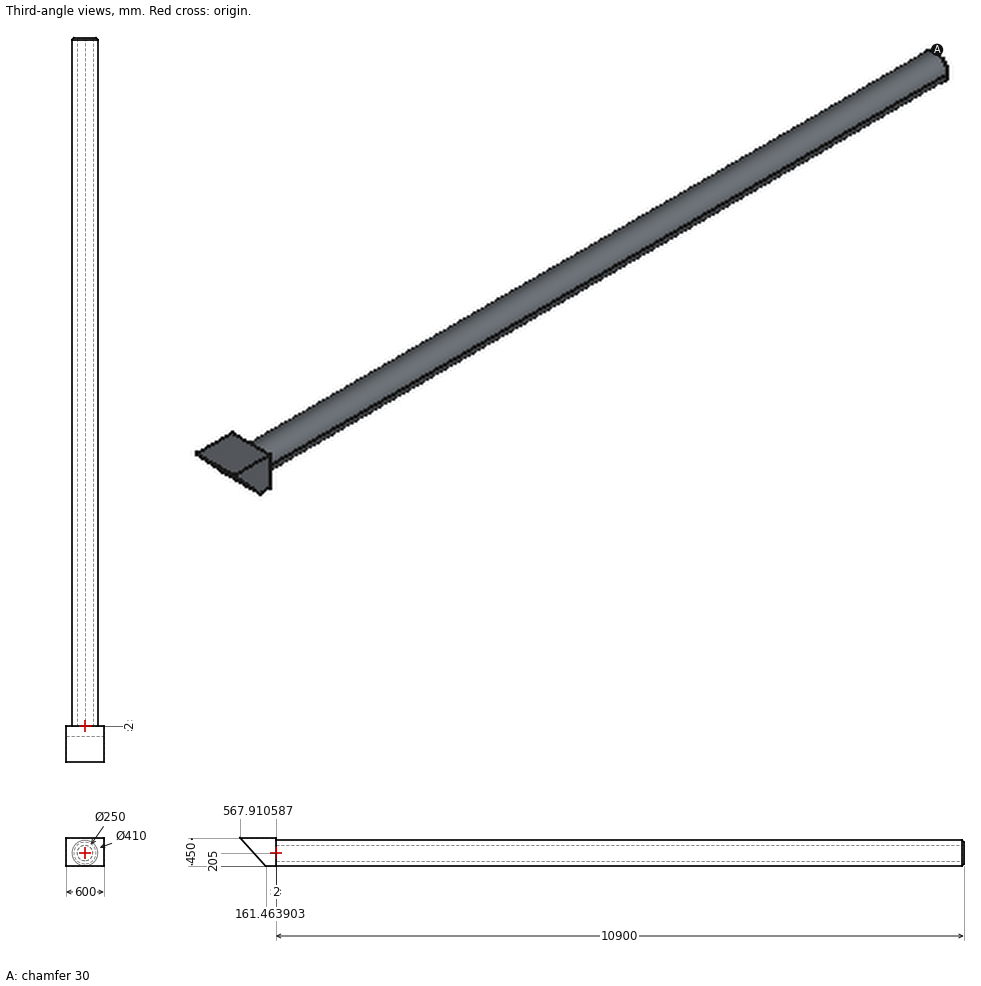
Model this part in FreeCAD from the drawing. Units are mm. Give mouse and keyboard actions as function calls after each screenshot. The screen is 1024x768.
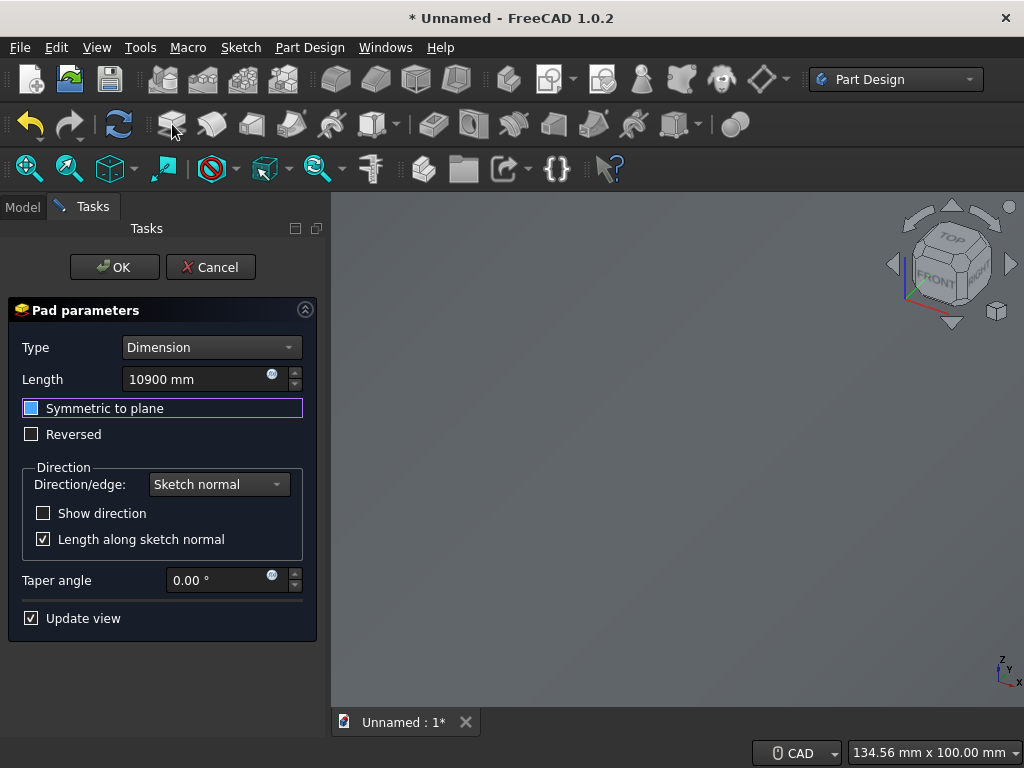
click(30, 434)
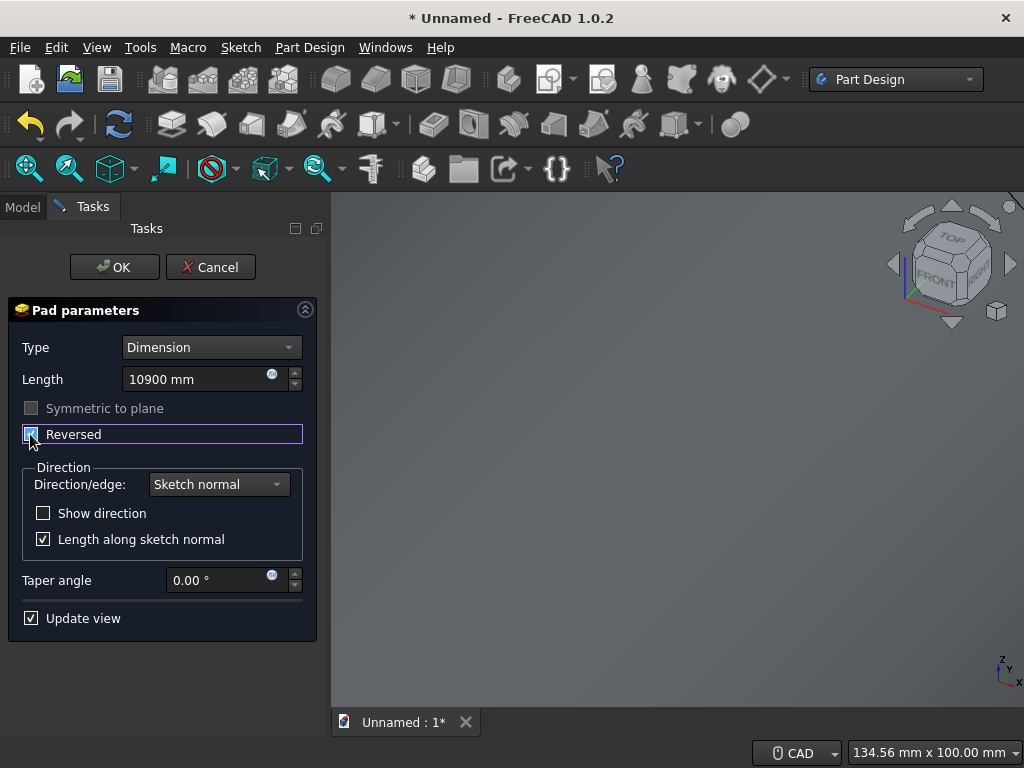
click(115, 267)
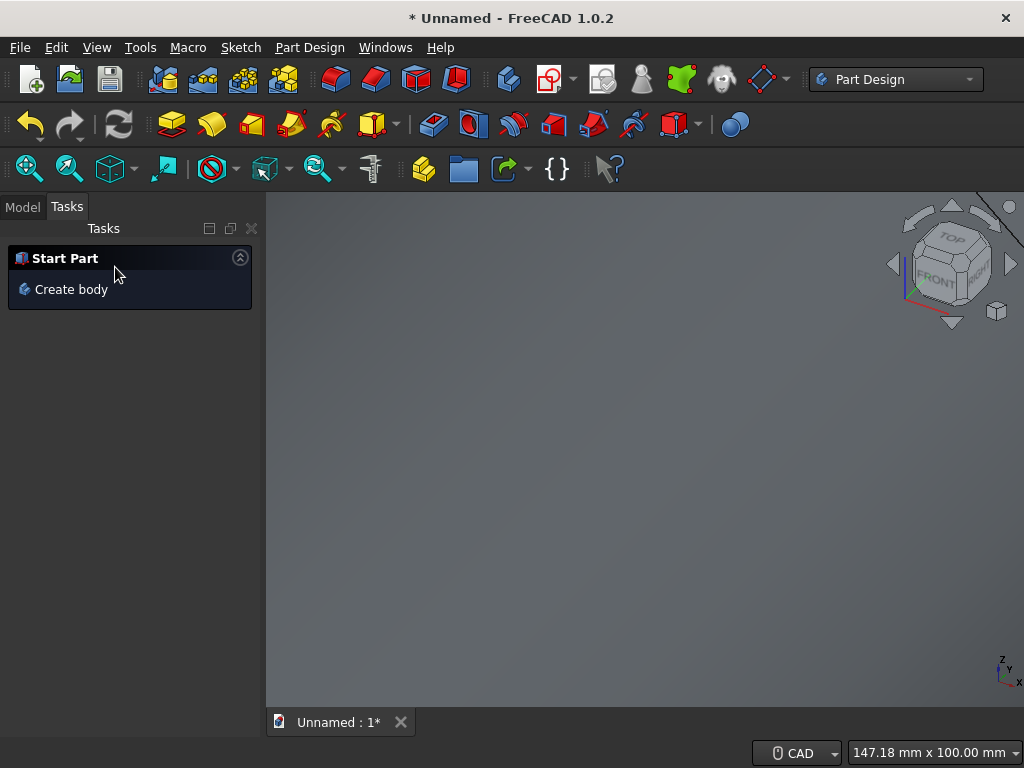
click(30, 170)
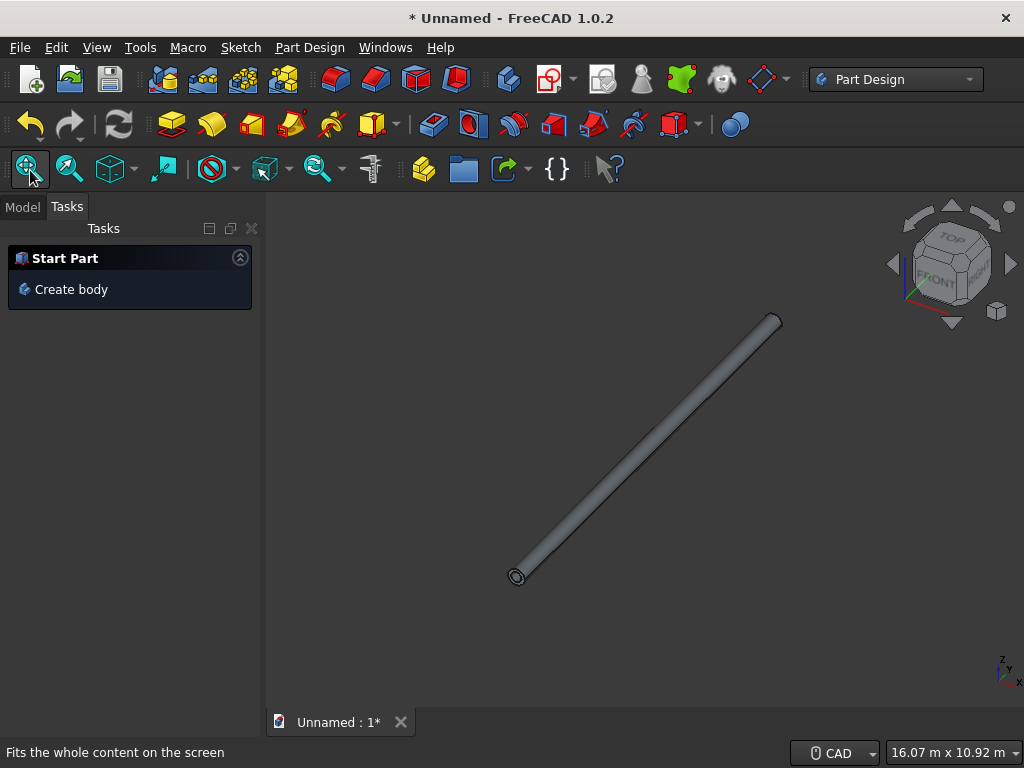
click(23, 206)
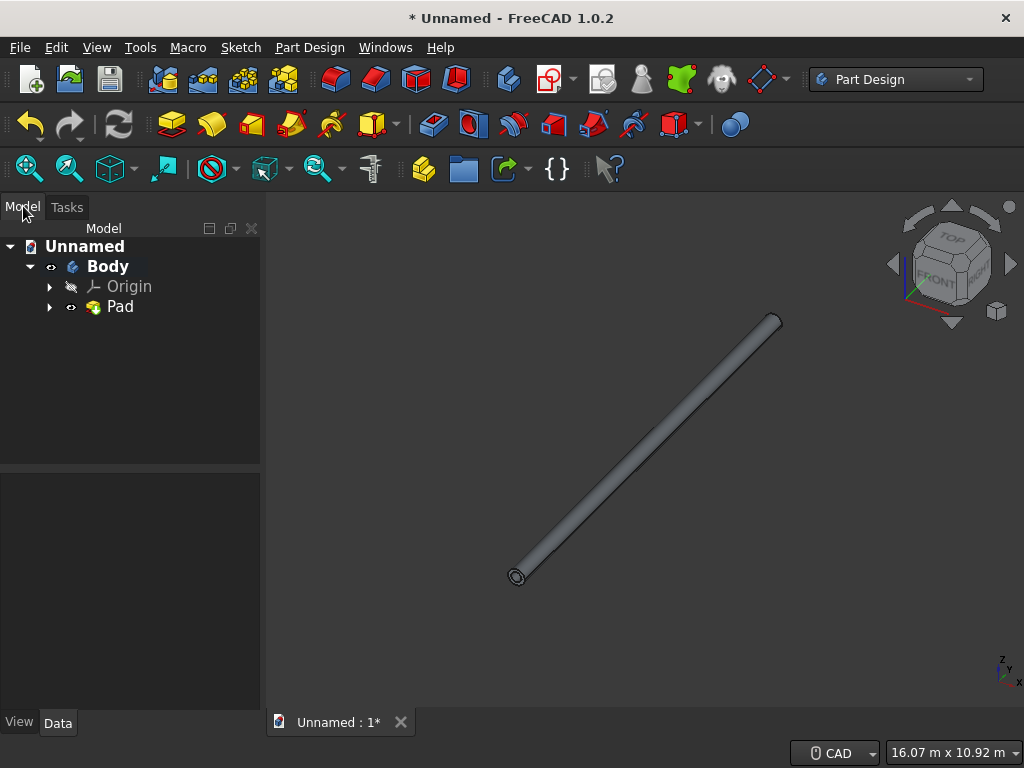
click(50, 287)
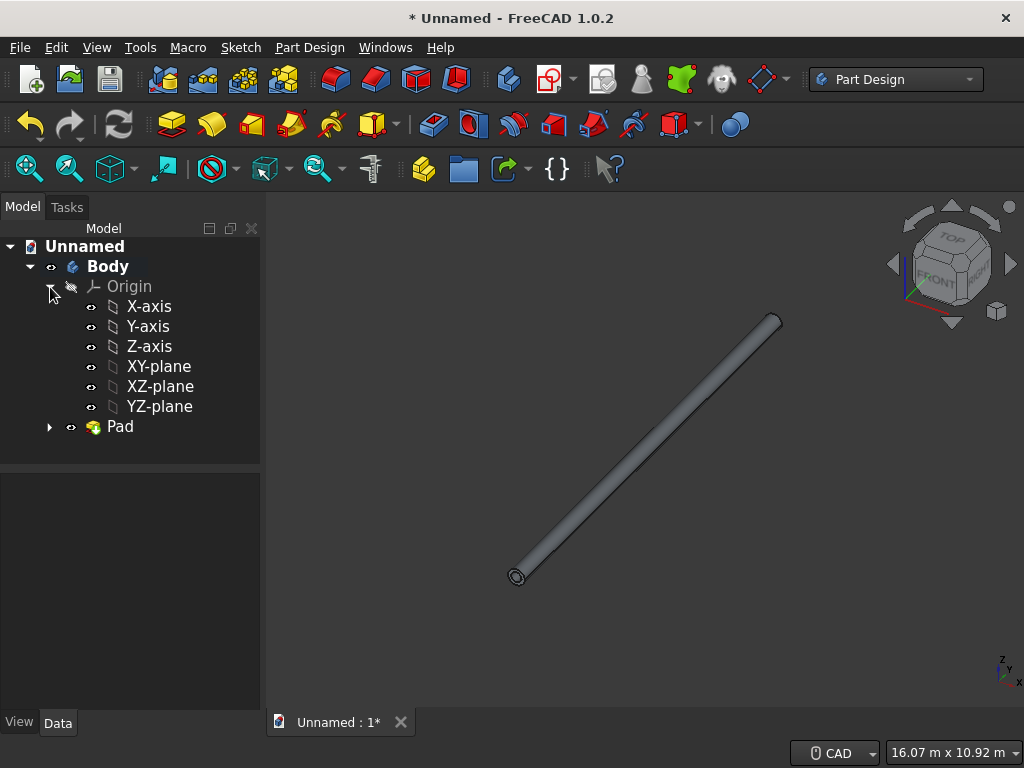
click(136, 387)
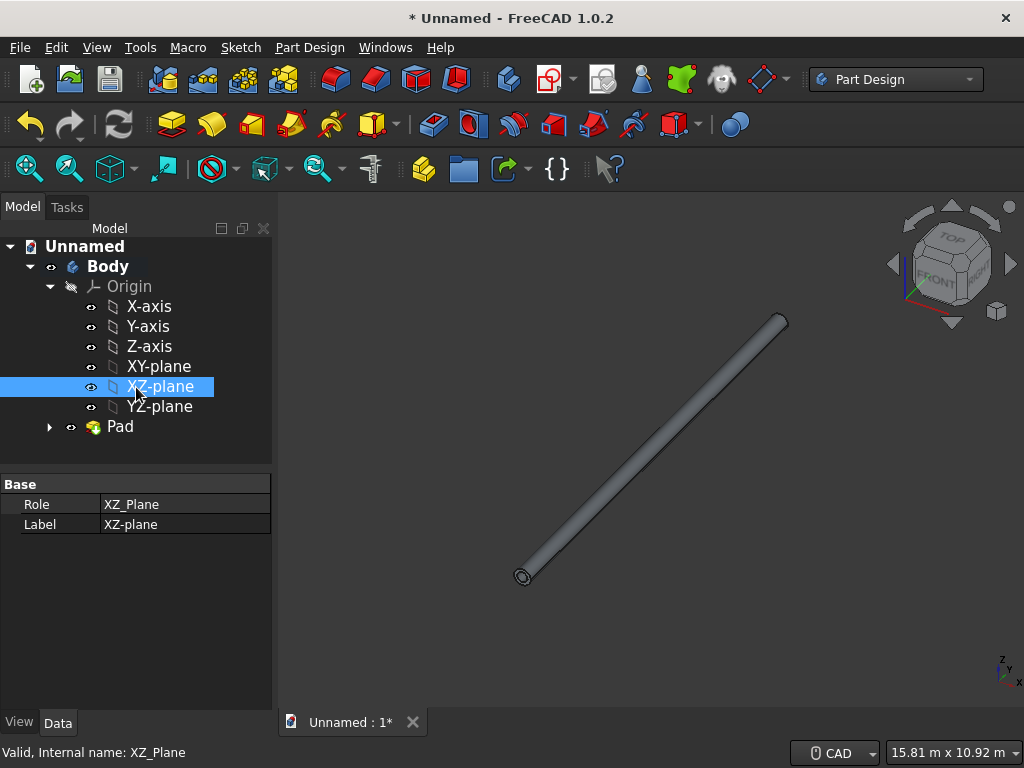
click(762, 80)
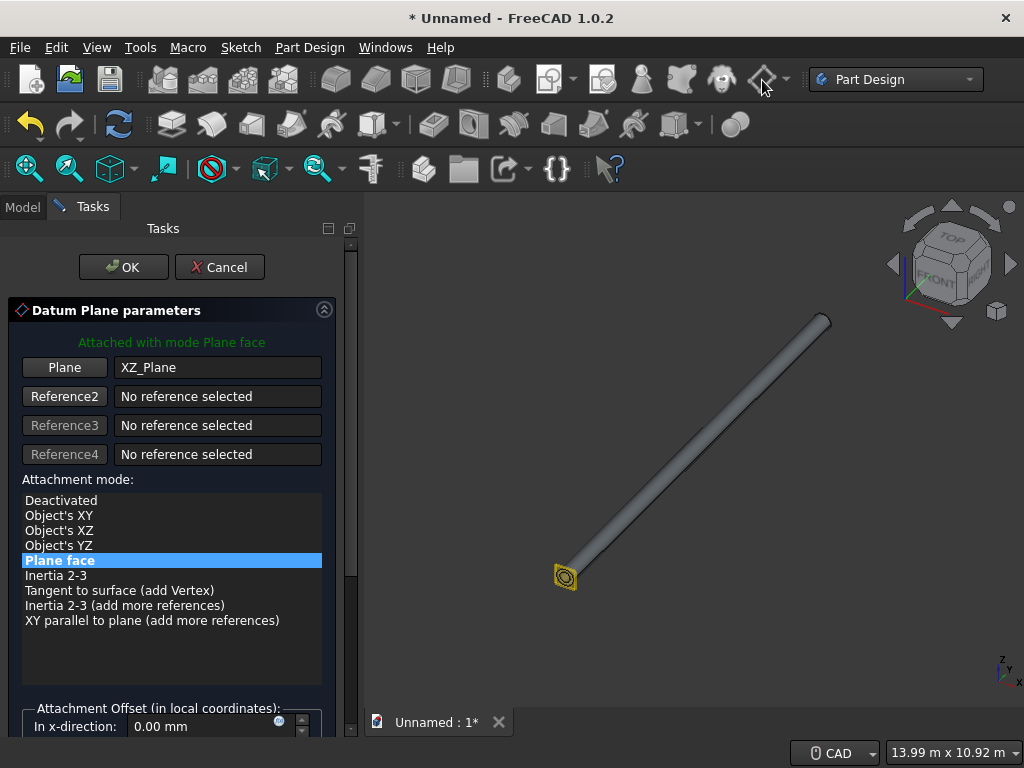
scroll(351, 487, down, 3)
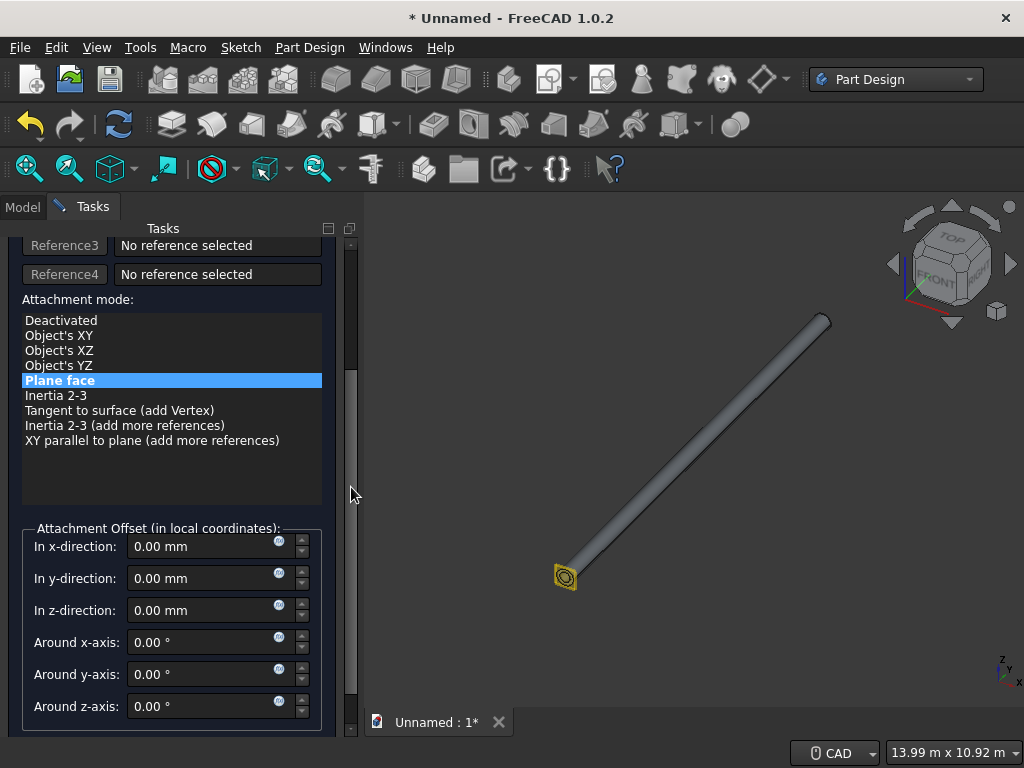
triple_click(210, 610)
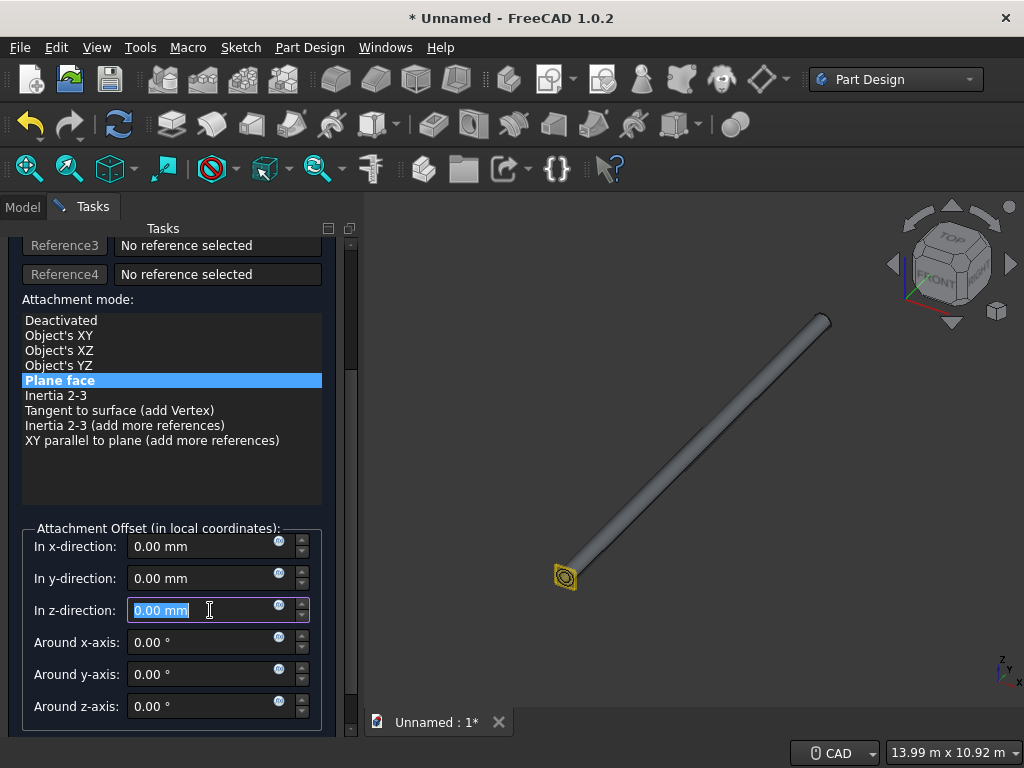
text(2)
key(Tab)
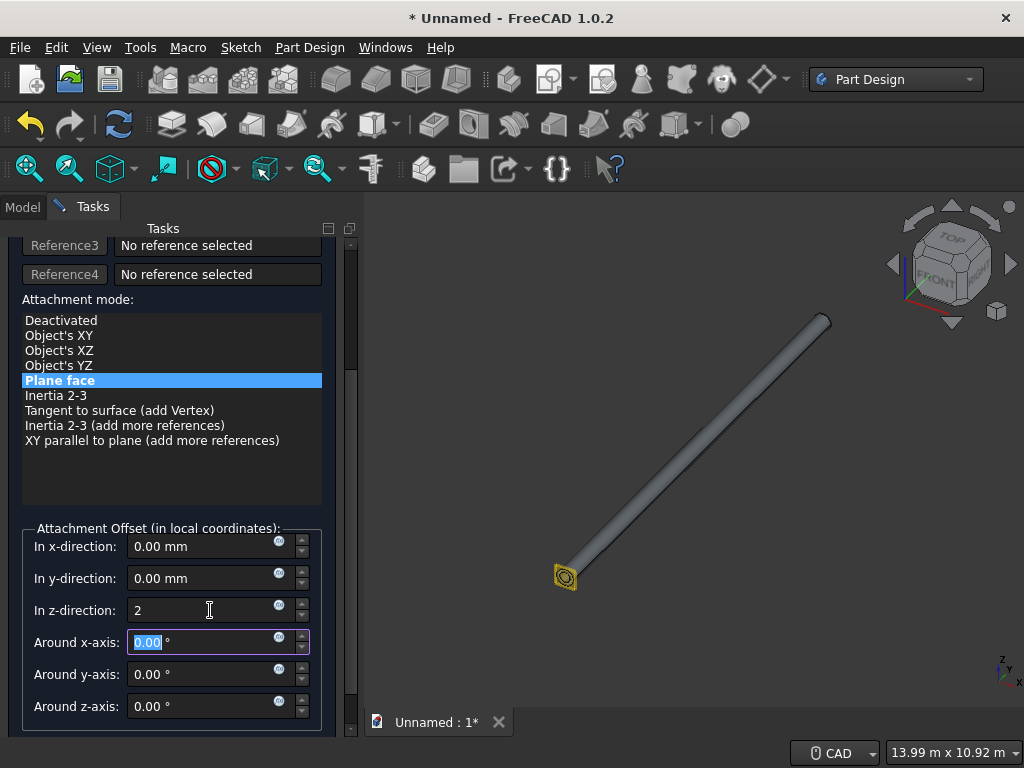
scroll(351, 487, up, 4)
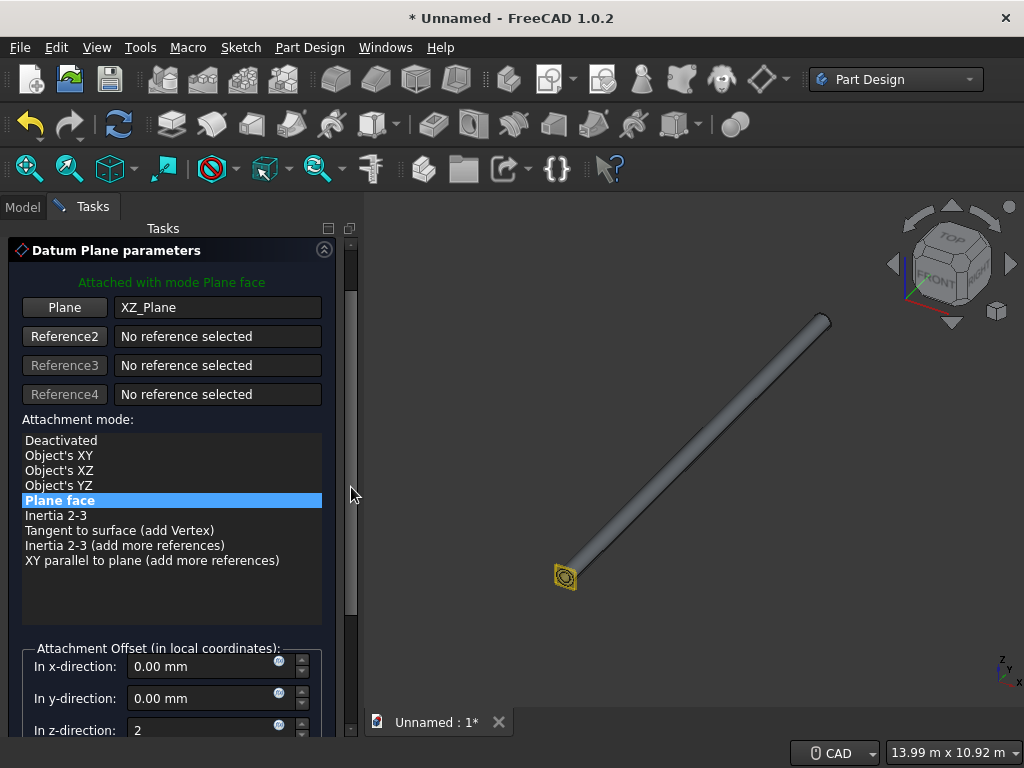
click(124, 267)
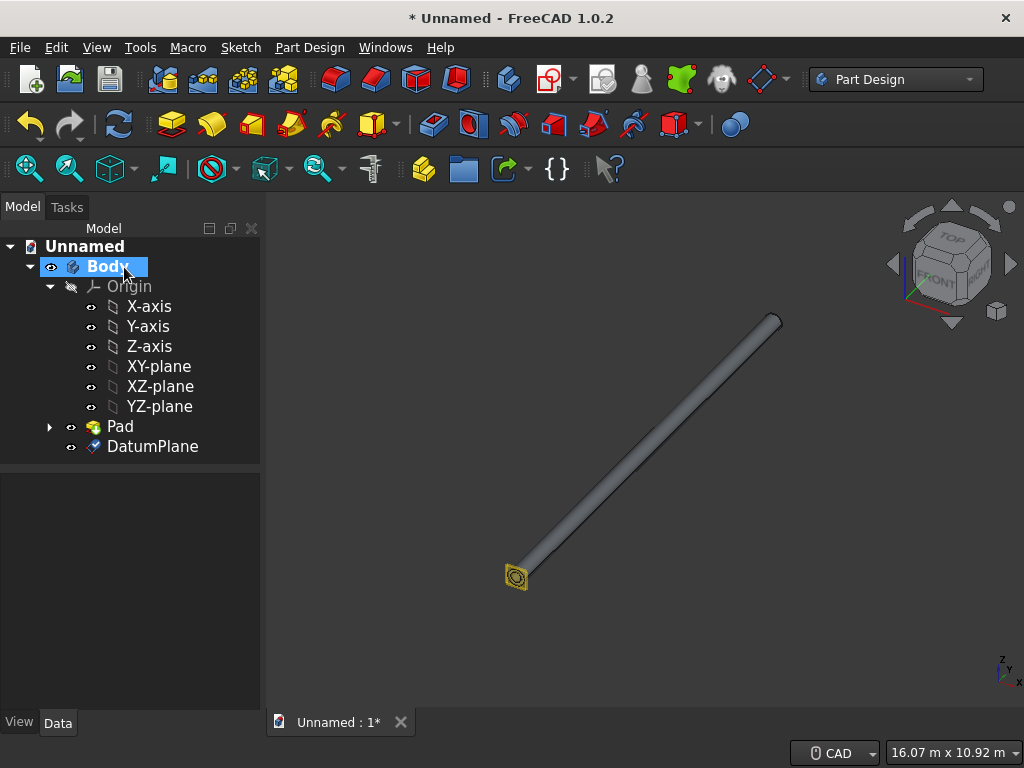
click(116, 447)